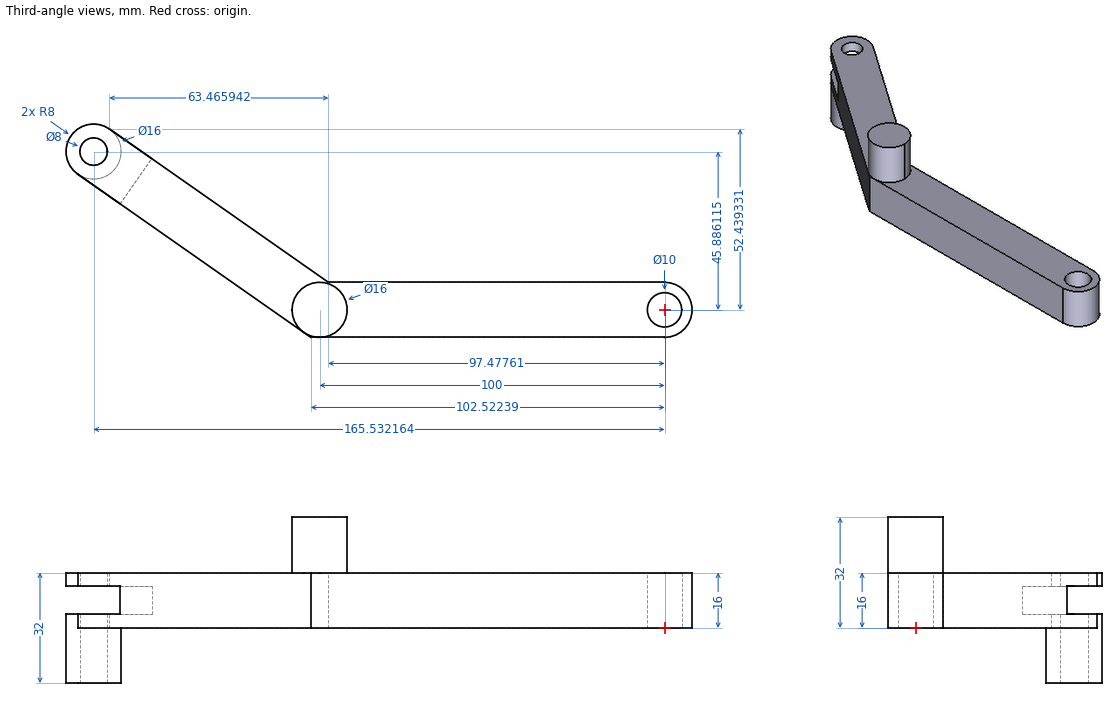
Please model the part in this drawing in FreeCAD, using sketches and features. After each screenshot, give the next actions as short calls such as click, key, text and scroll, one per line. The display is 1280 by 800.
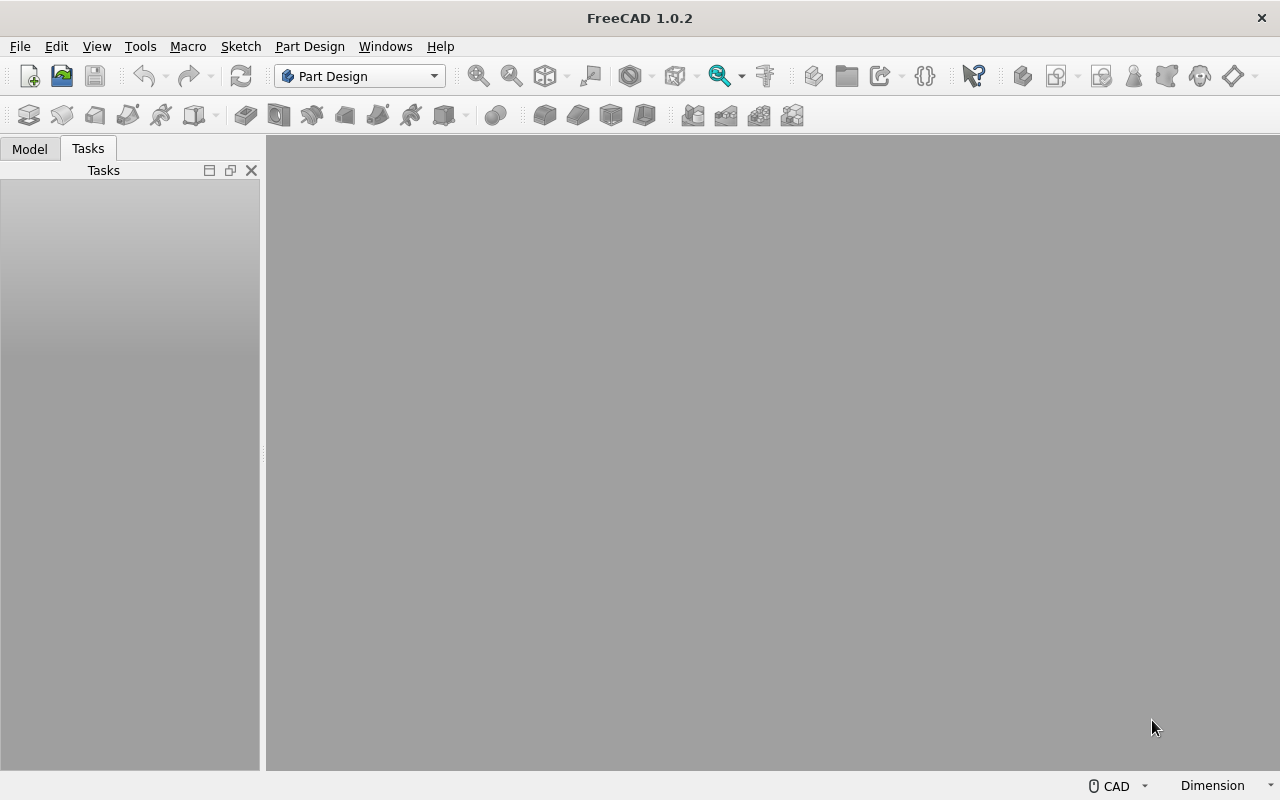
click(29, 76)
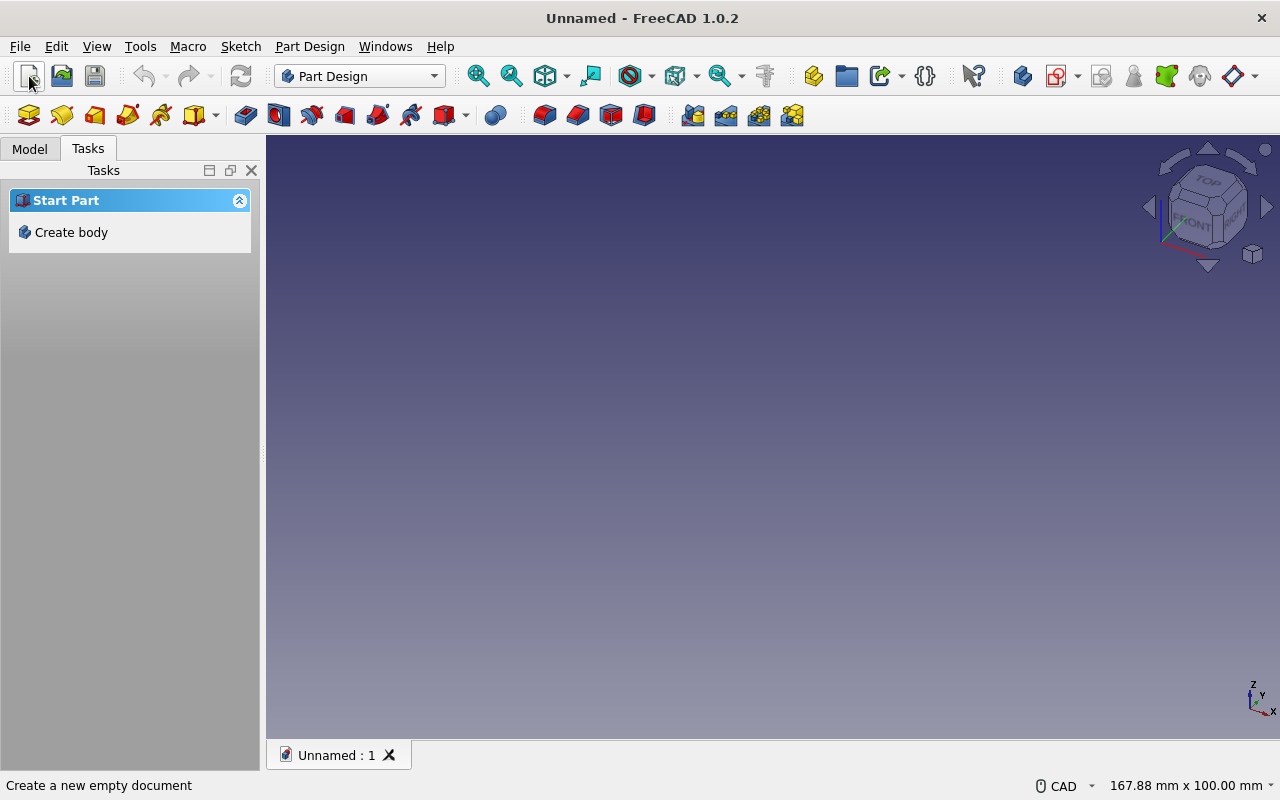
click(1056, 76)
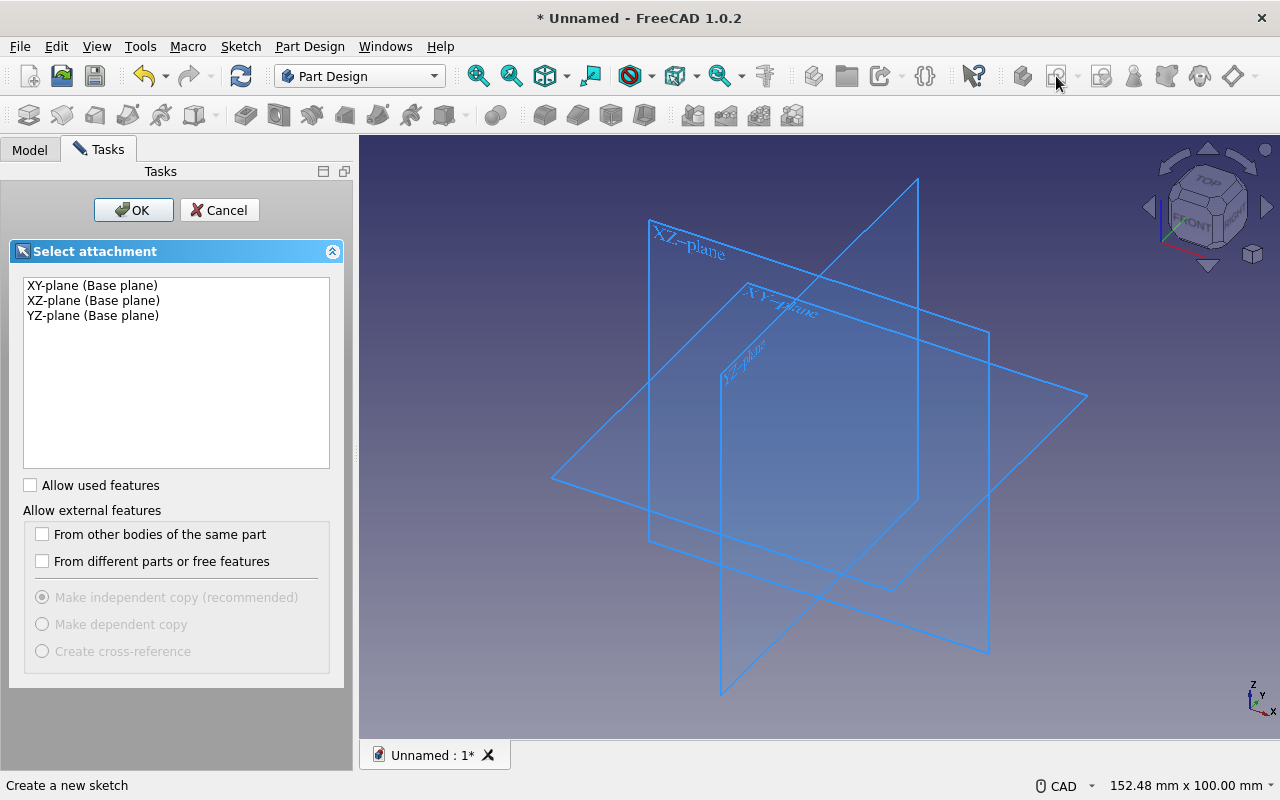
click(84, 286)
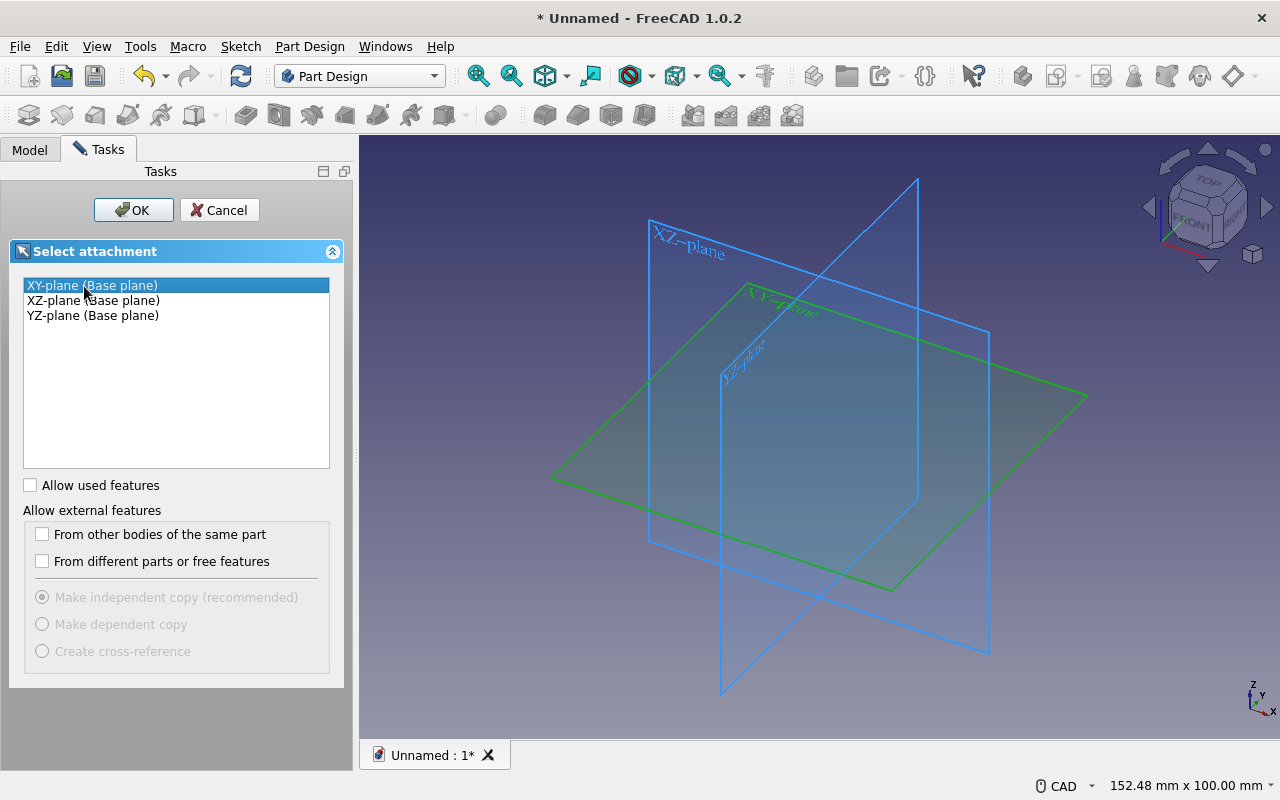
click(134, 210)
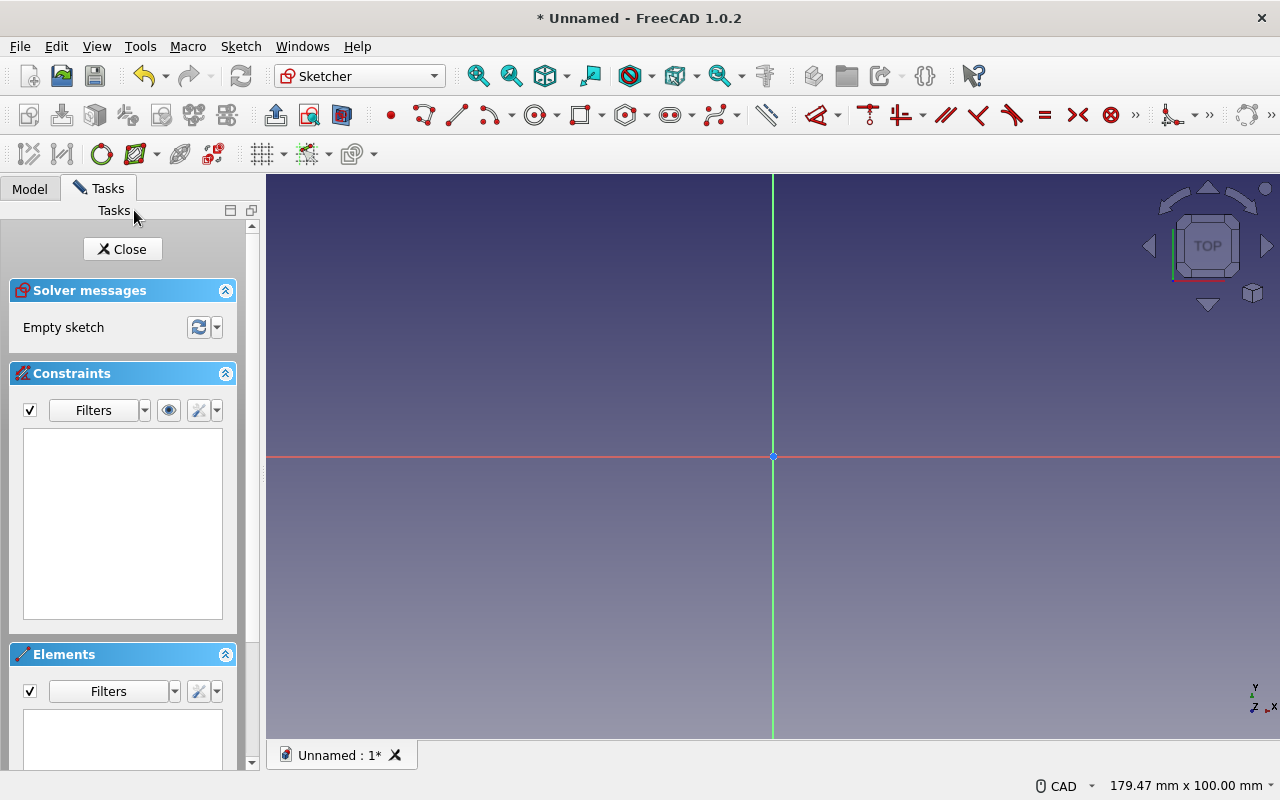
scroll(1115, 609, down, 3)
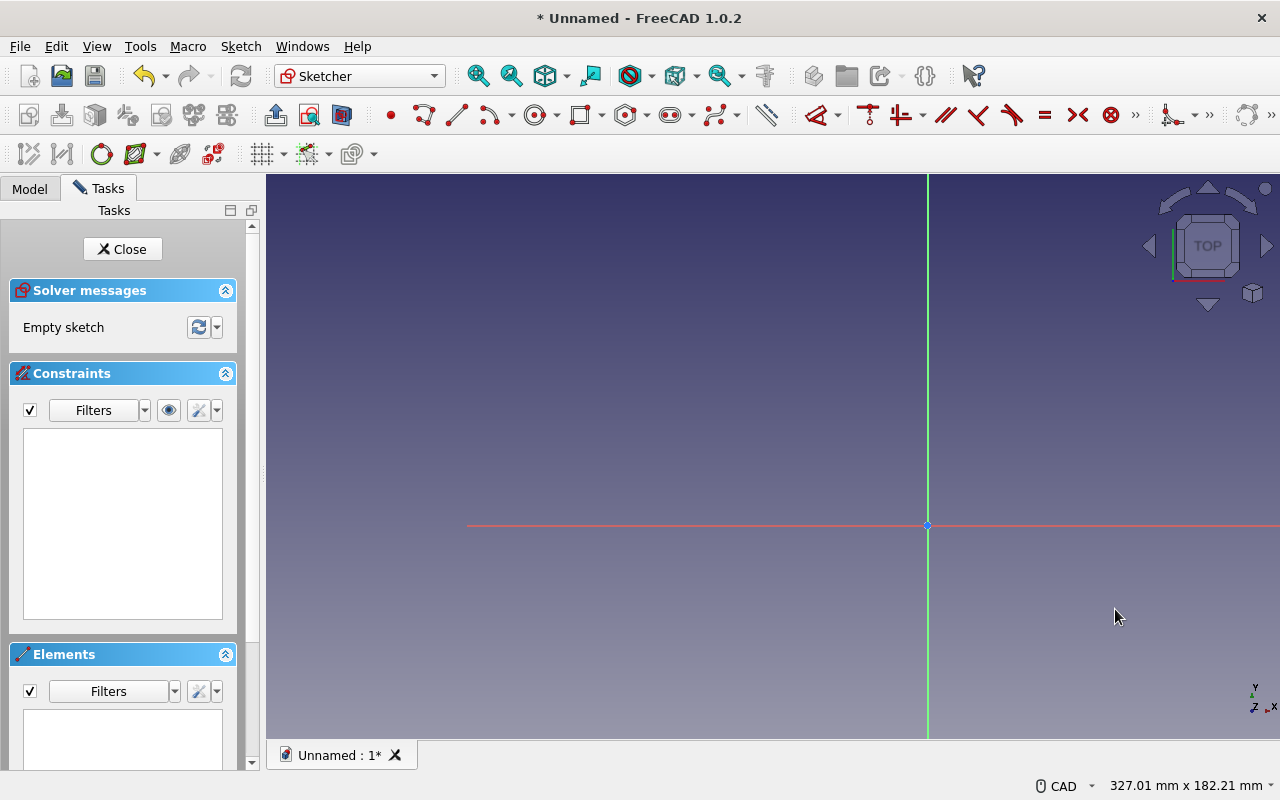
click(424, 116)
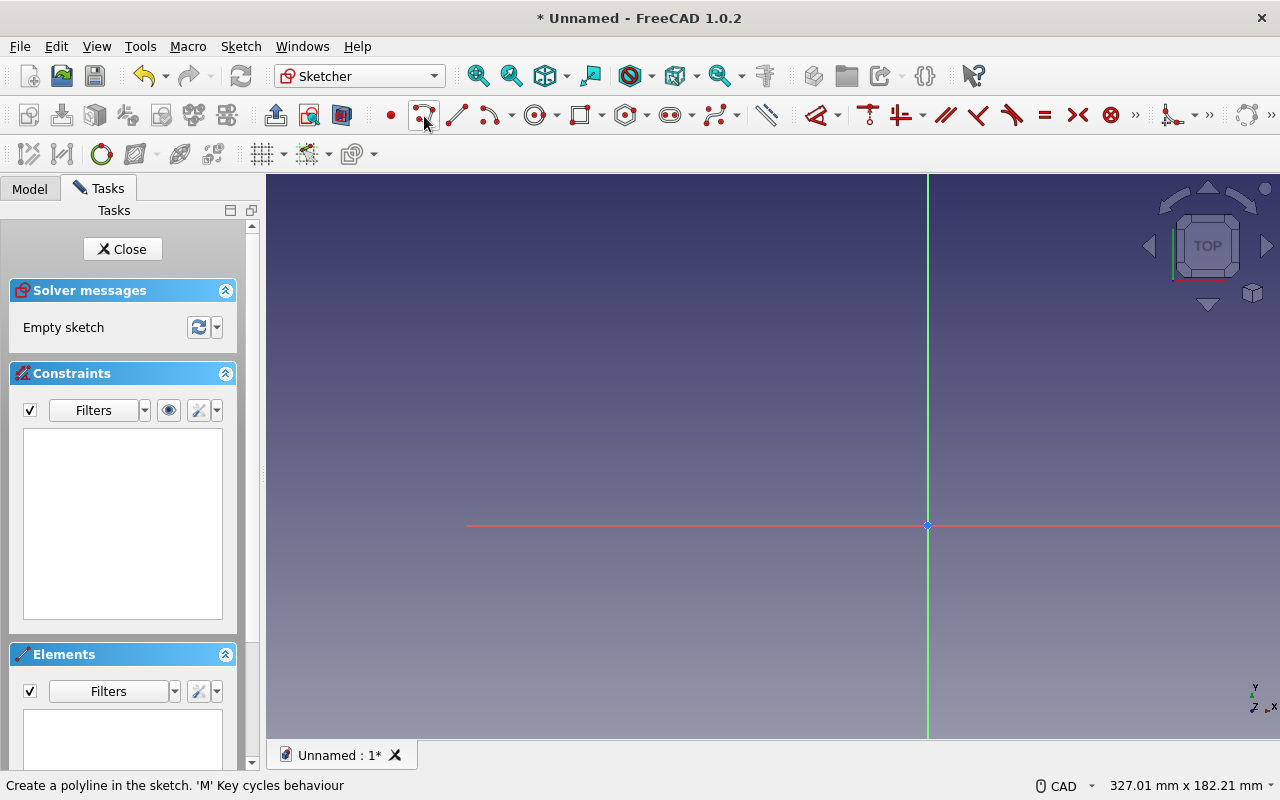
click(928, 501)
click(625, 501)
click(429, 363)
right_click(429, 363)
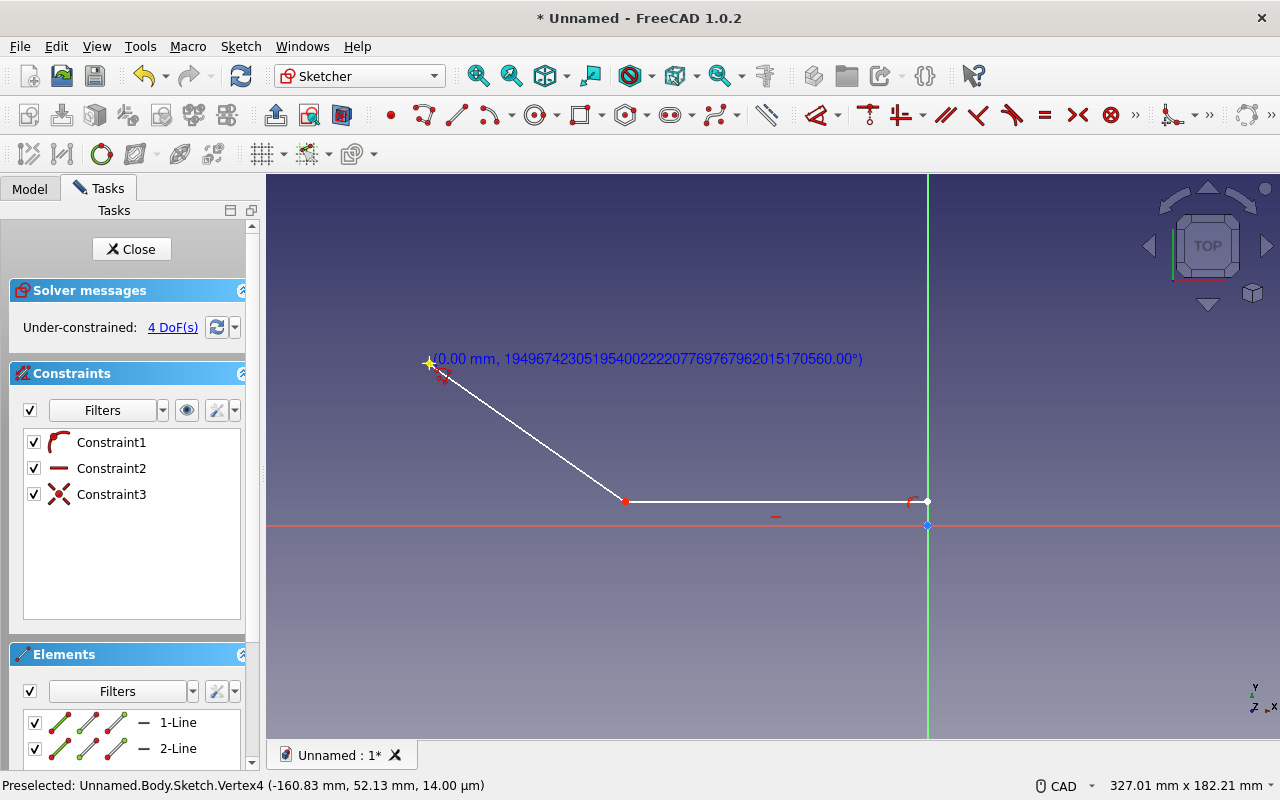
click(400, 404)
click(610, 550)
click(928, 550)
right_click(928, 550)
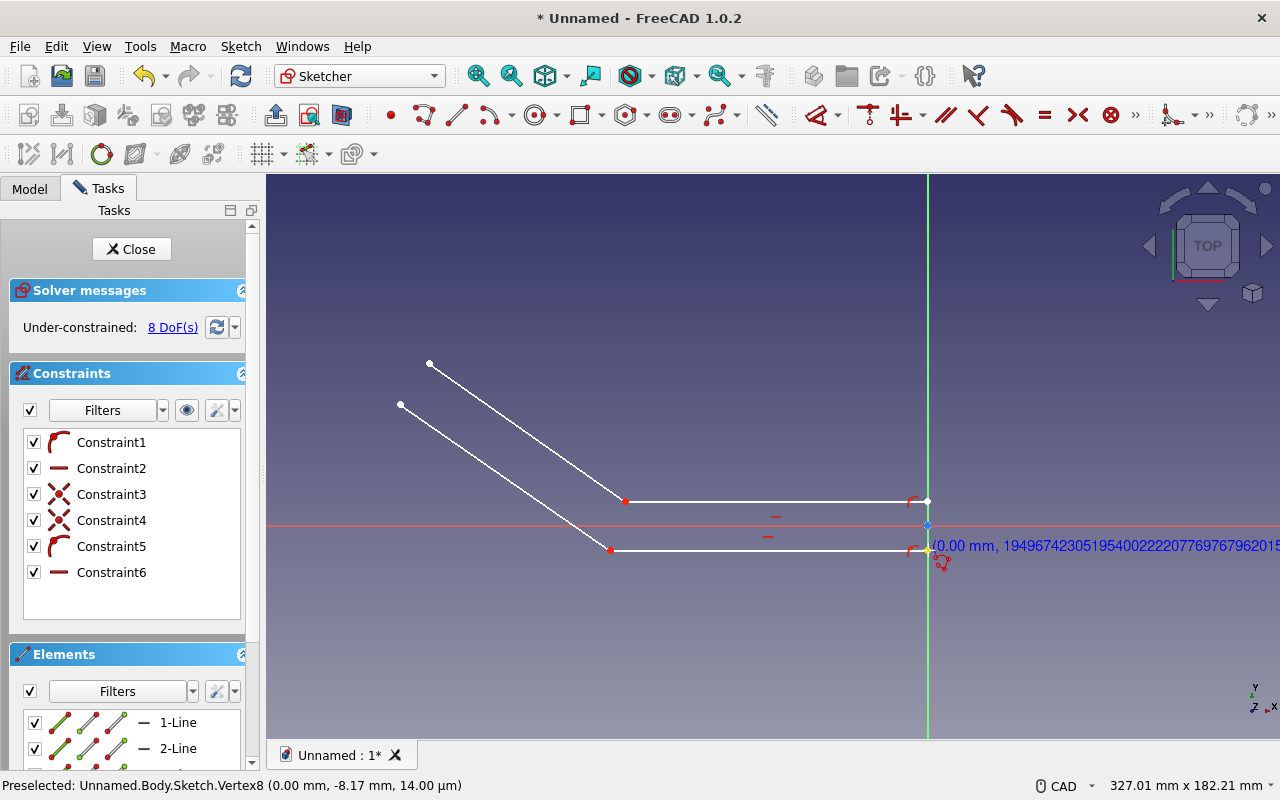
key(g)
key(3)
key(a)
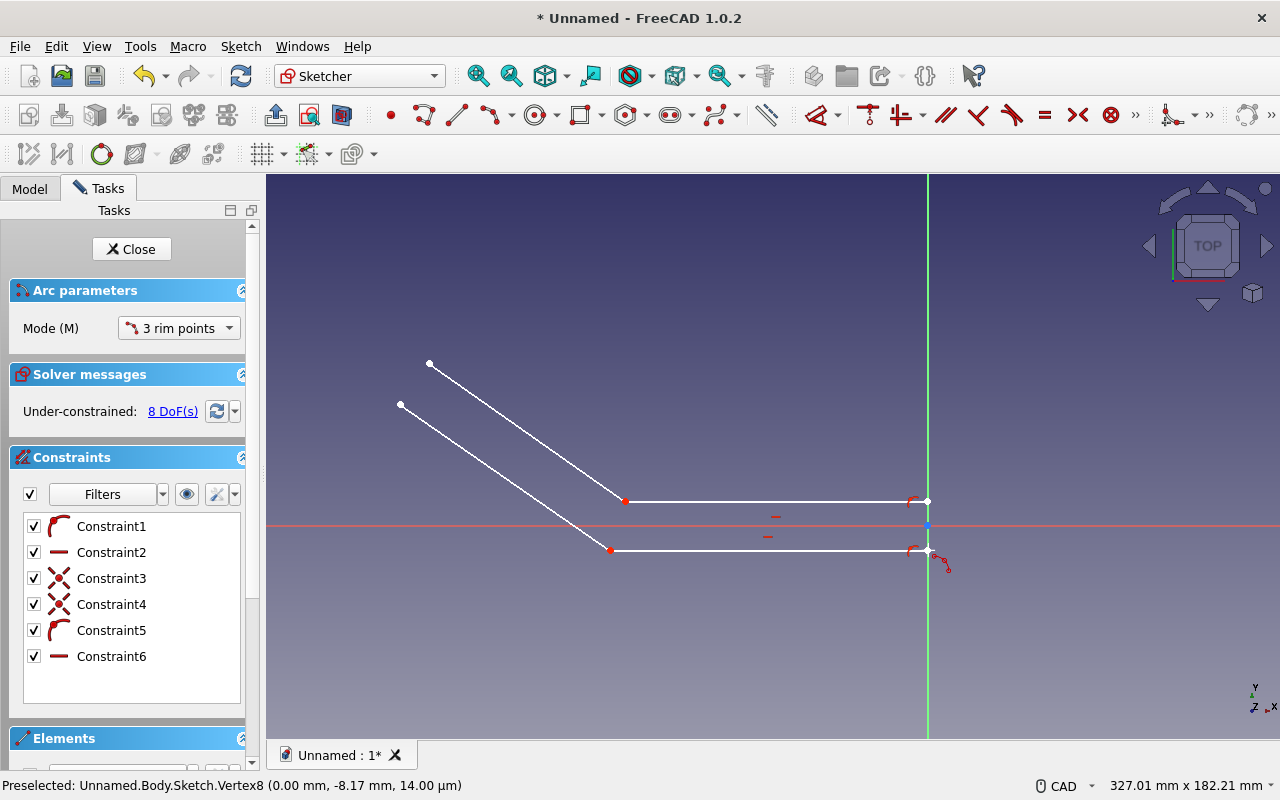
click(429, 364)
click(400, 405)
click(394, 369)